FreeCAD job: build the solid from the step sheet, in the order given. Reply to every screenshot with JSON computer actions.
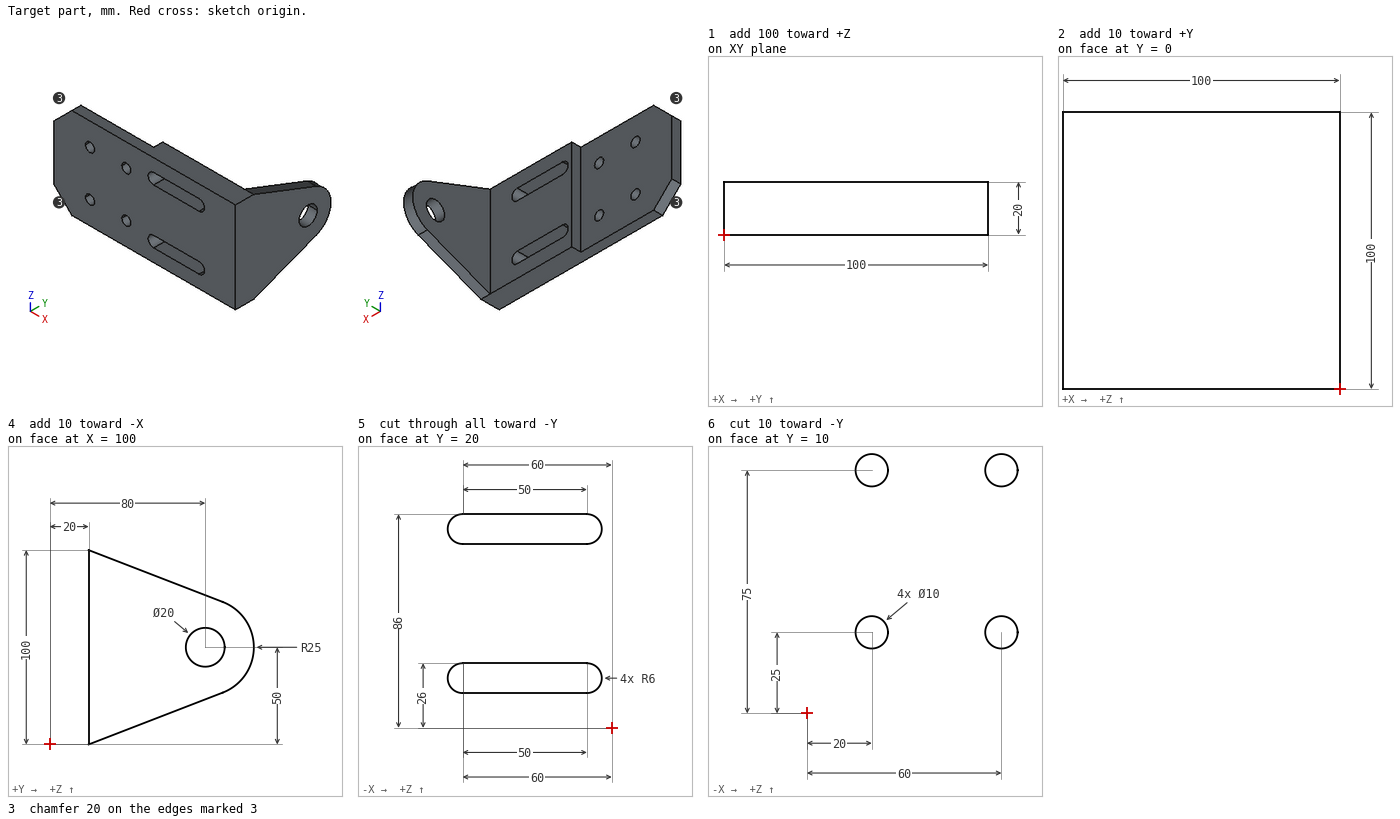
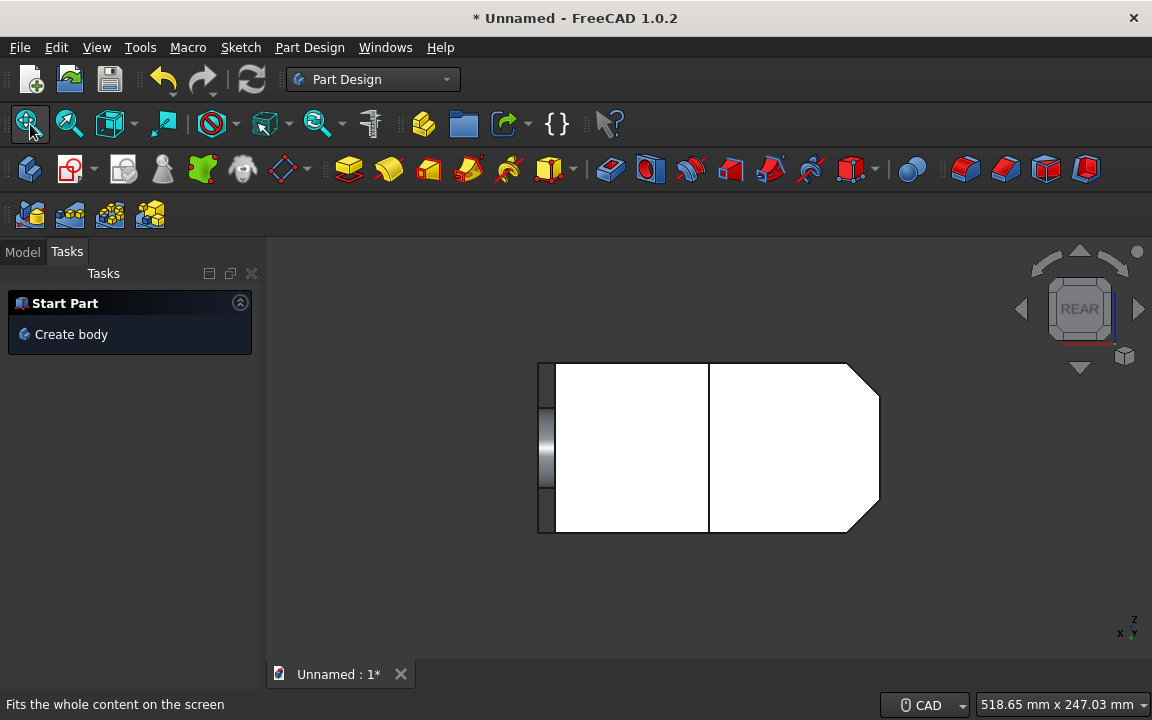
{"action": "left_click", "coordinate": [30, 124]}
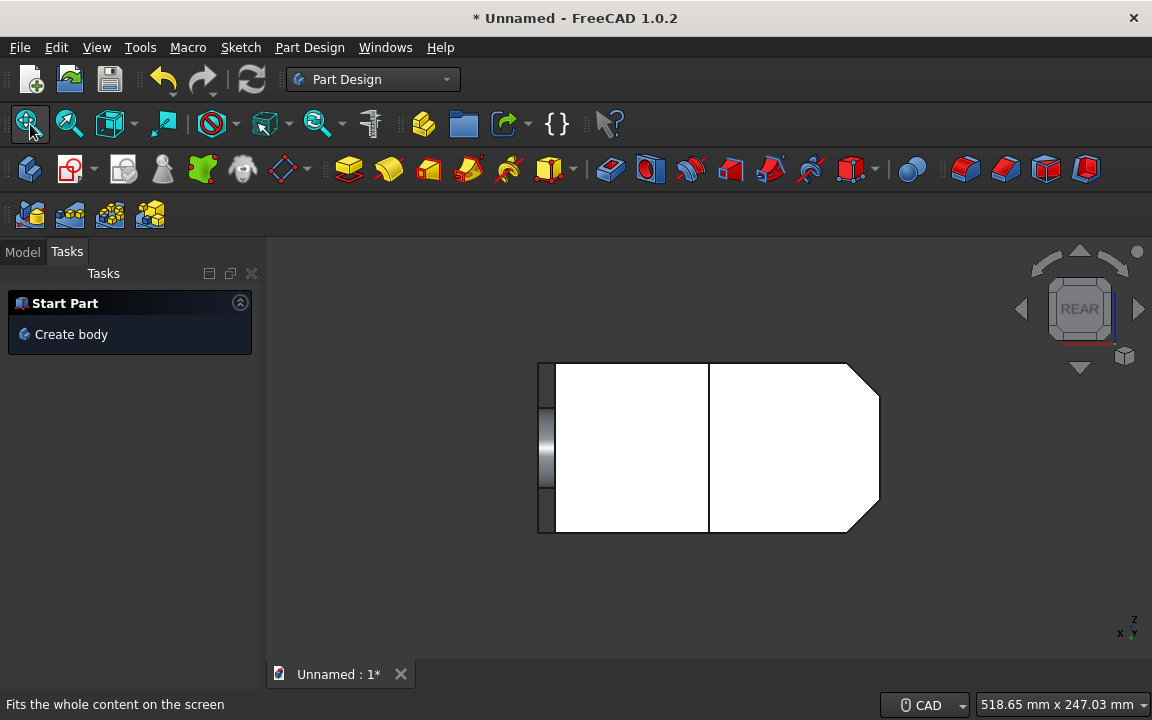
{"action": "left_click", "coordinate": [632, 447]}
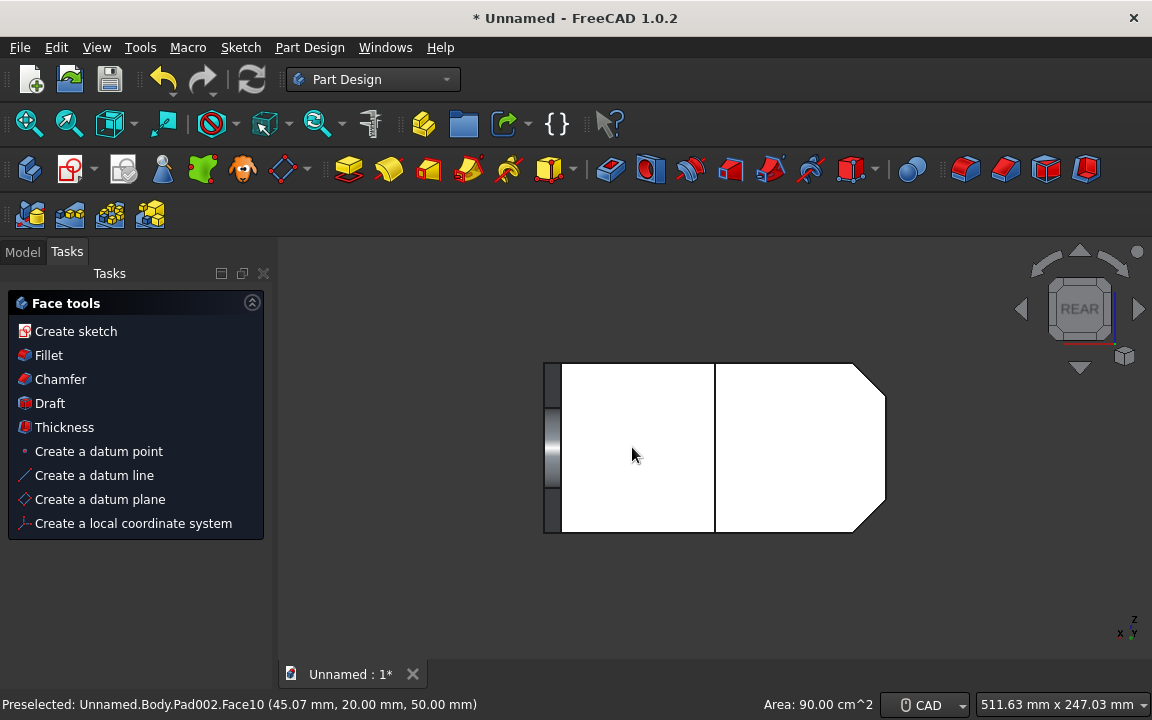
{"action": "left_click", "coordinate": [70, 170]}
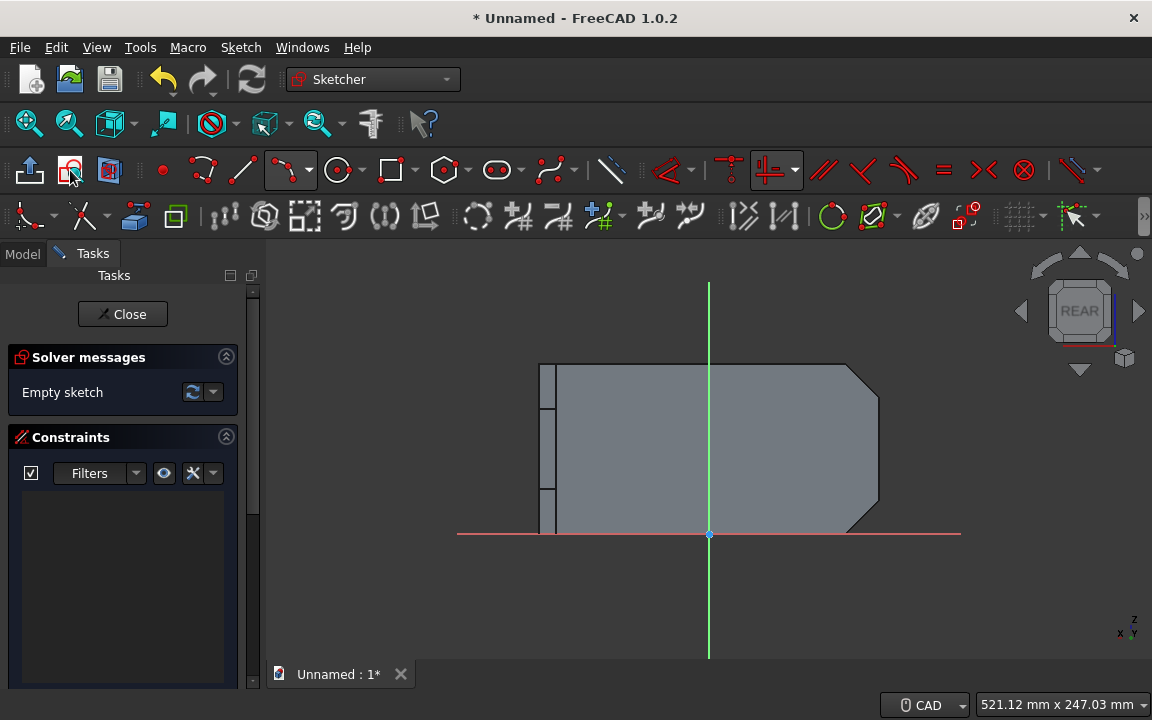
{"action": "left_click", "coordinate": [110, 170]}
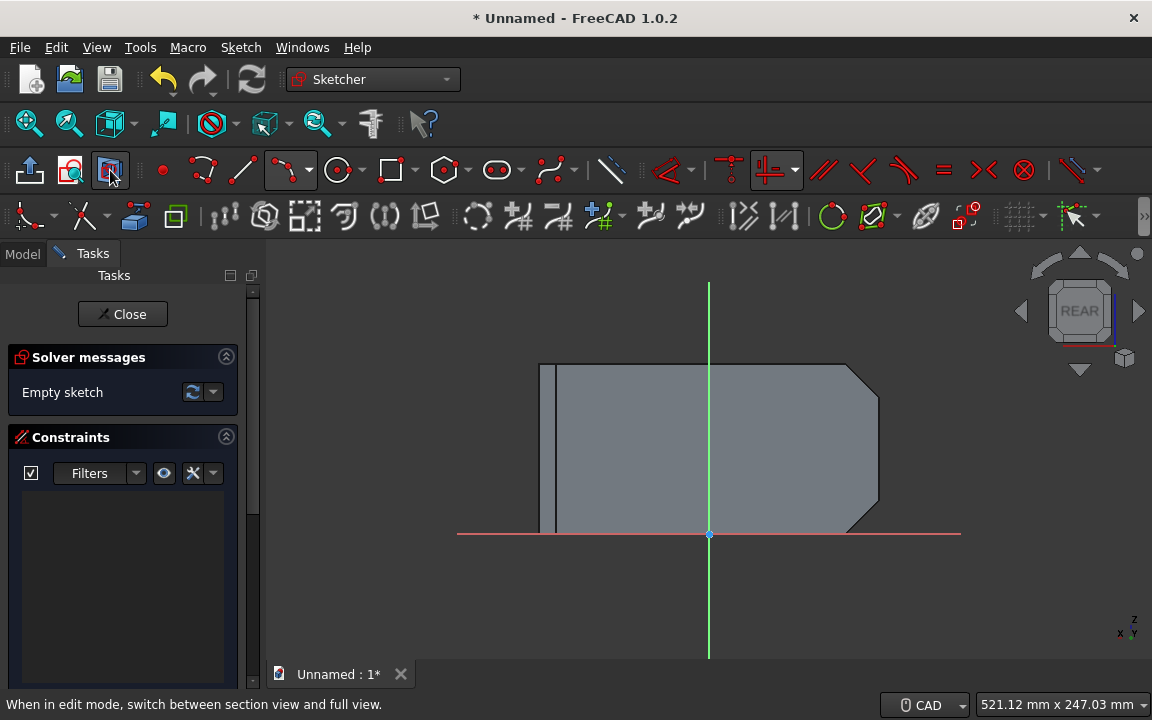
{"action": "scroll", "coordinate": [668, 475], "scroll_direction": "up", "scroll_amount": 3}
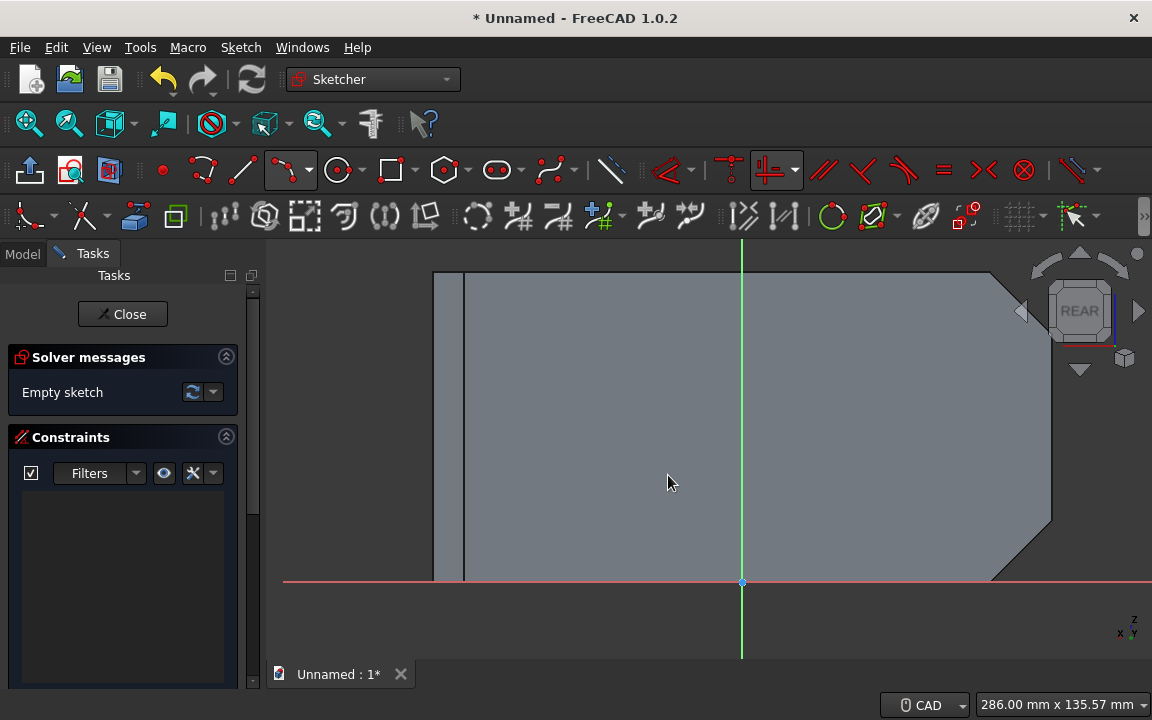
{"action": "left_click", "coordinate": [498, 170]}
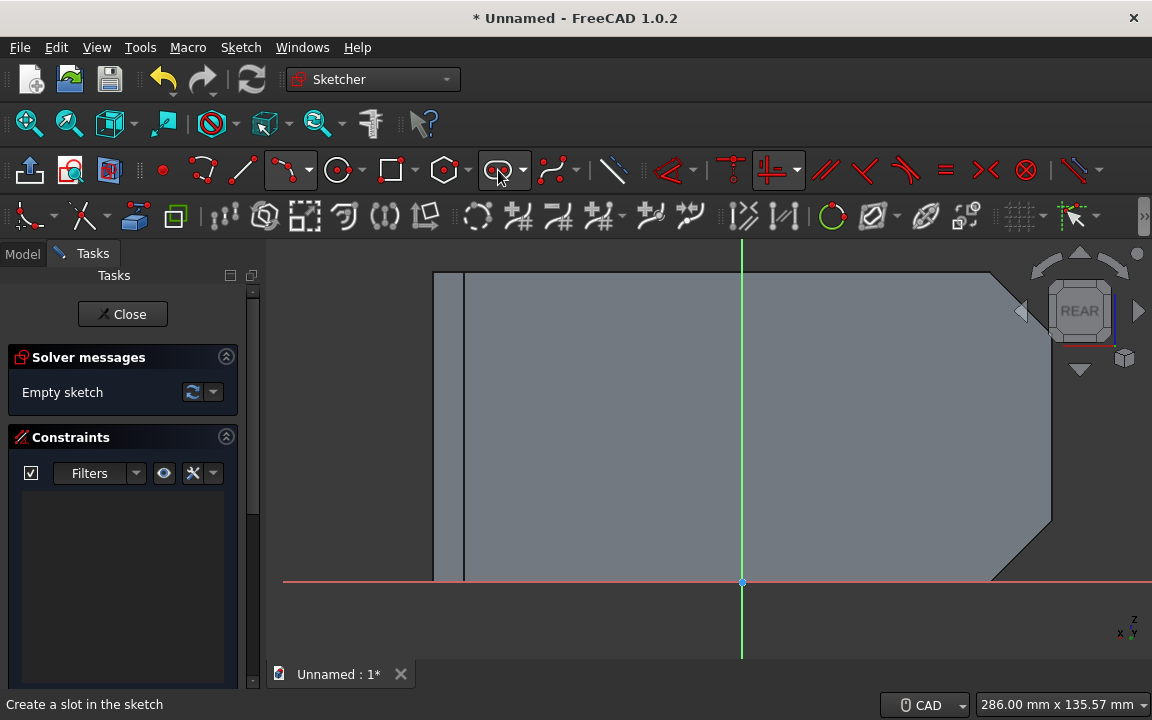
{"action": "left_click", "coordinate": [556, 520]}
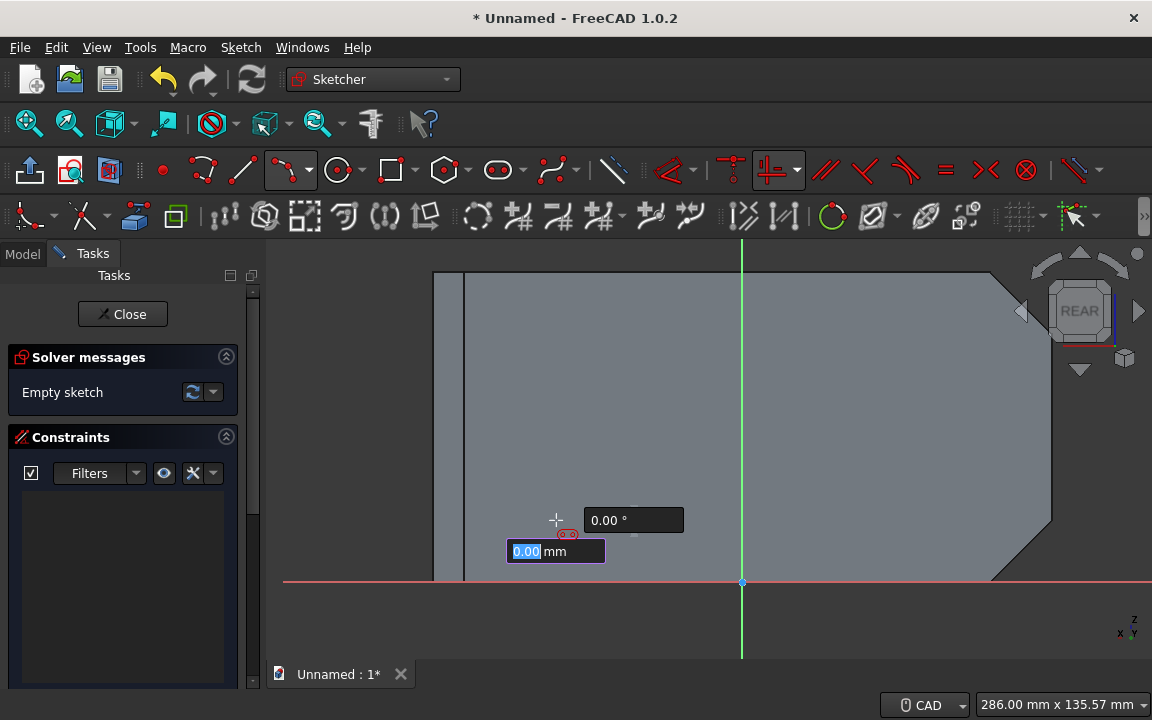
{"action": "left_click", "coordinate": [711, 520]}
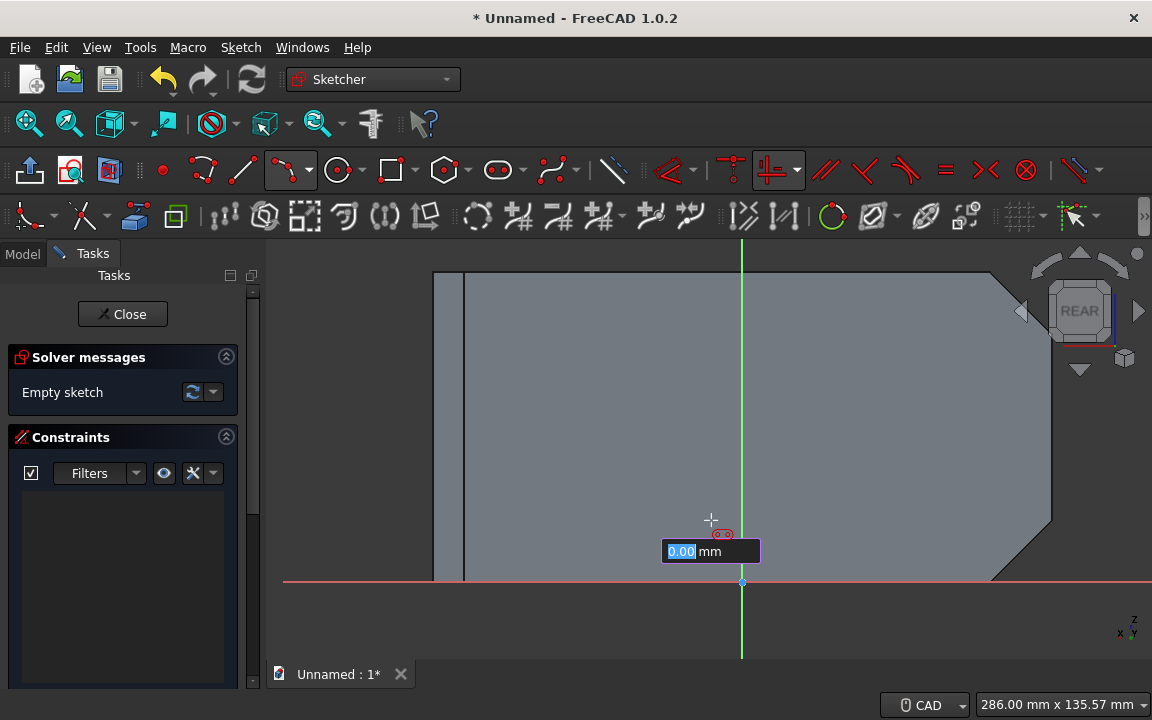
{"action": "left_click", "coordinate": [634, 539]}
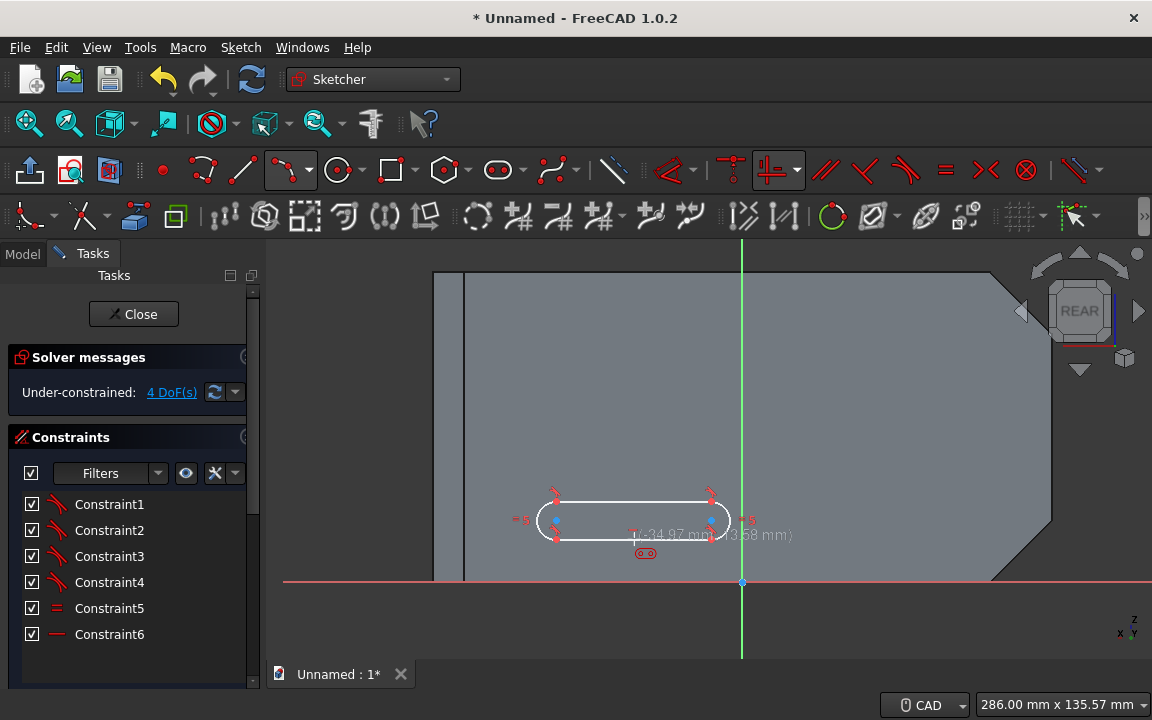
{"action": "left_click", "coordinate": [556, 334]}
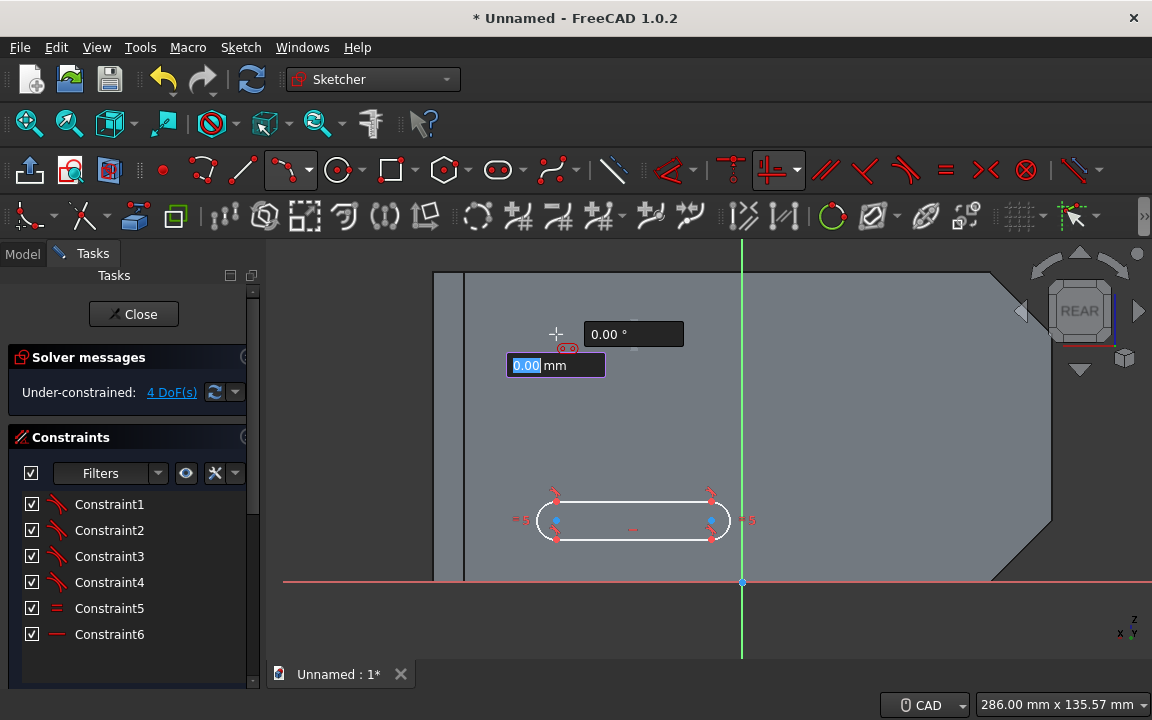
{"action": "left_click", "coordinate": [711, 334]}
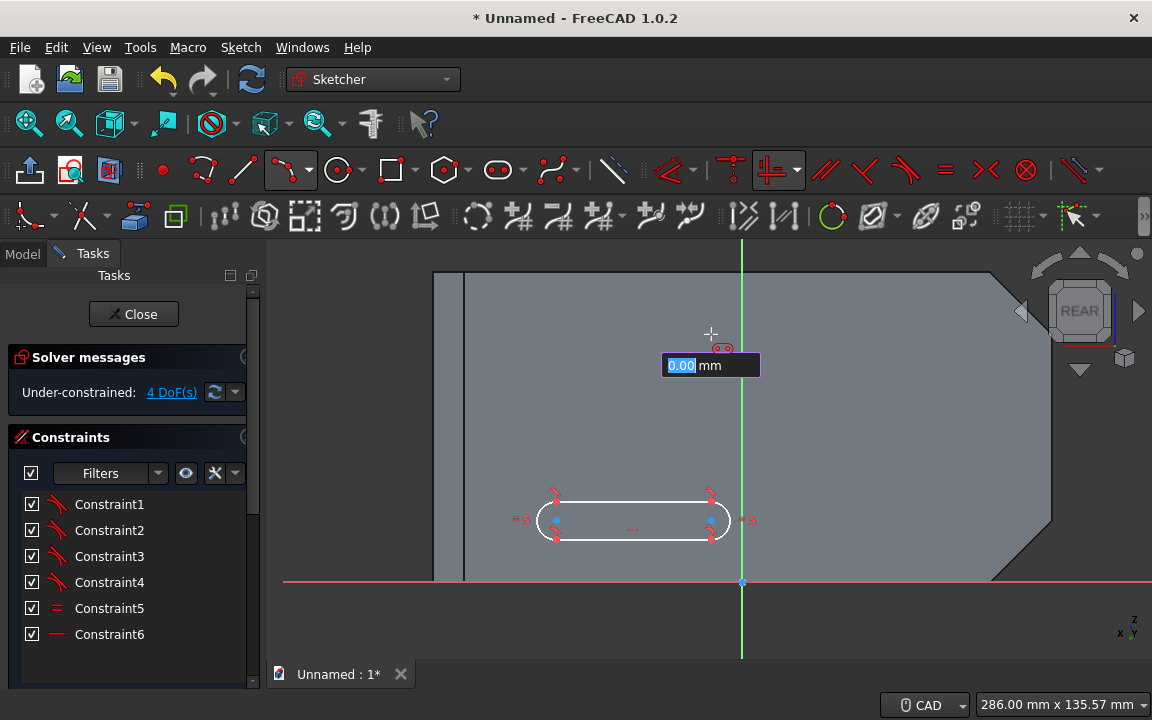
{"action": "left_click", "coordinate": [634, 316]}
{"action": "key", "text": "Escape"}